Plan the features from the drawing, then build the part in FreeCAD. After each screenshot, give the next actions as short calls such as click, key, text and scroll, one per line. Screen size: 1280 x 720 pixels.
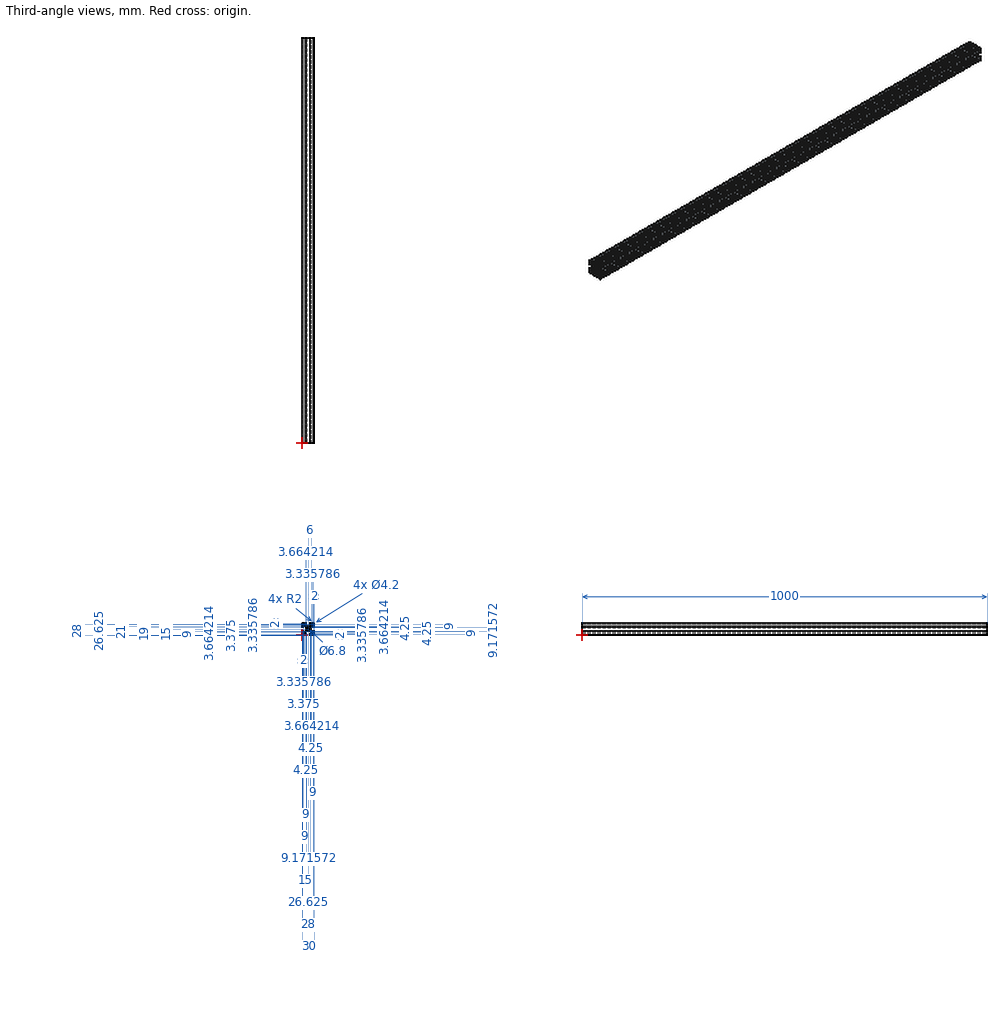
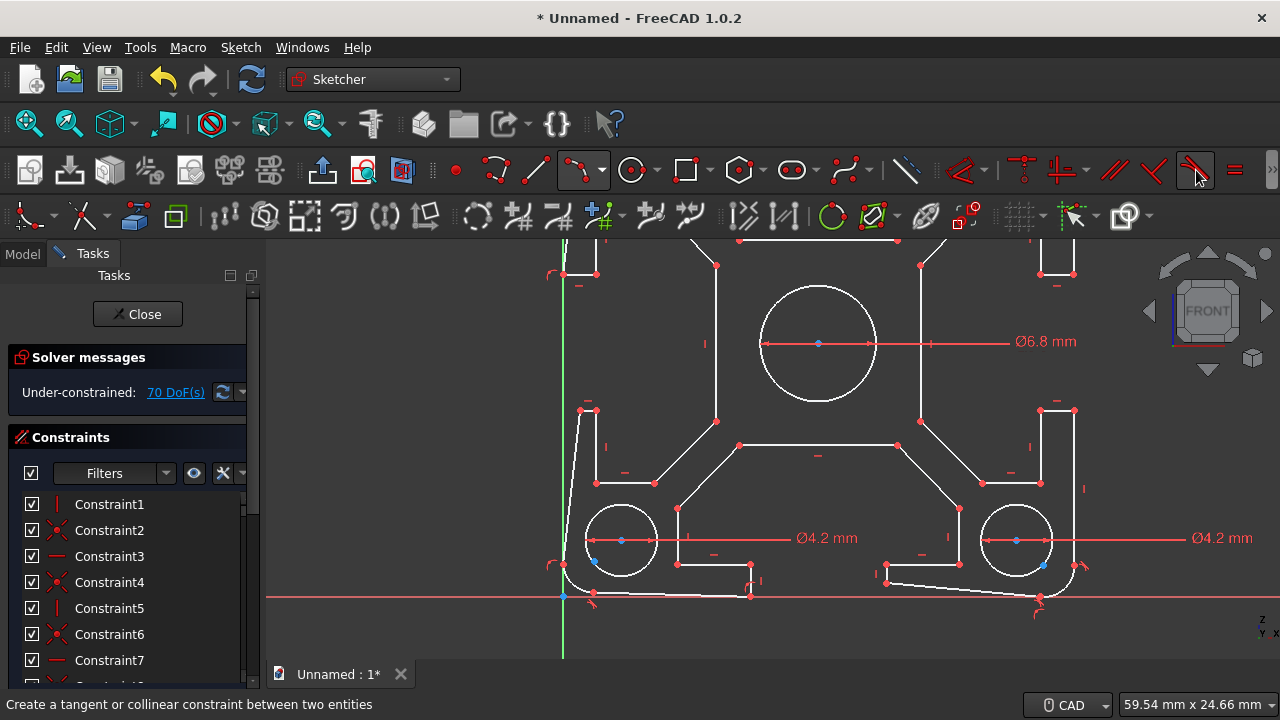
click(575, 457)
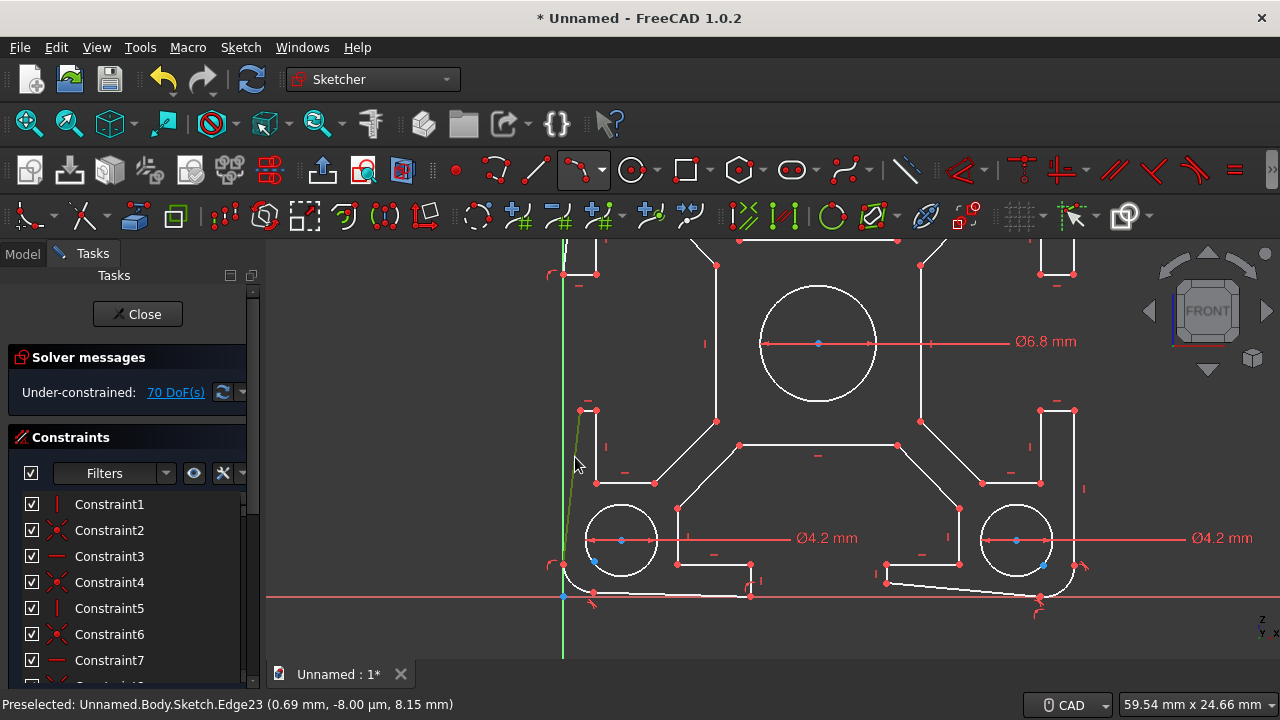
scroll(573, 584, up, 2)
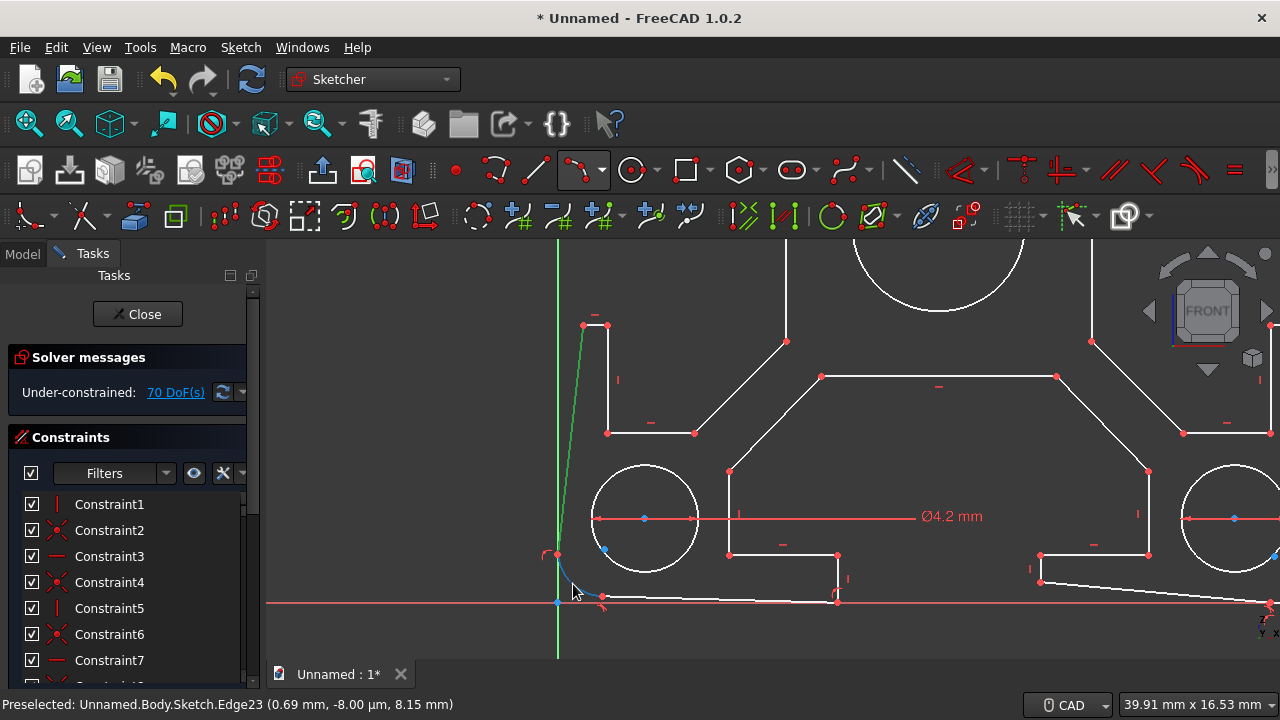
click(573, 584)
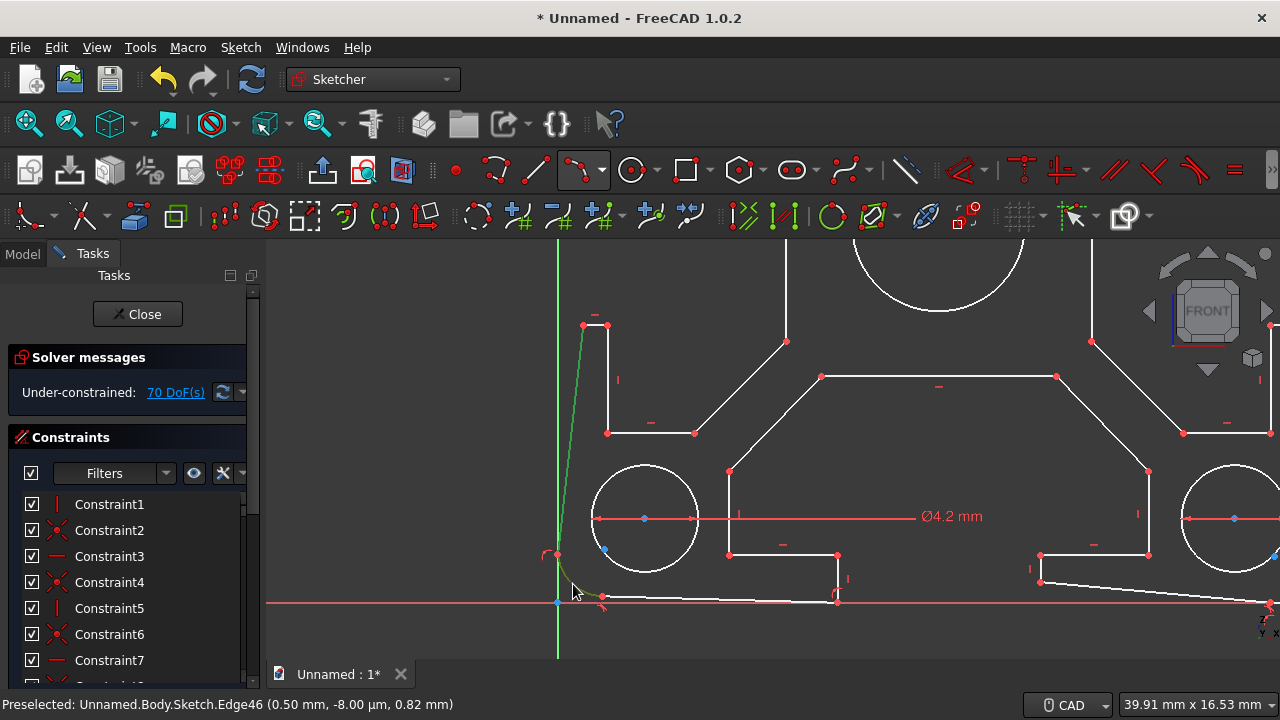
key(t)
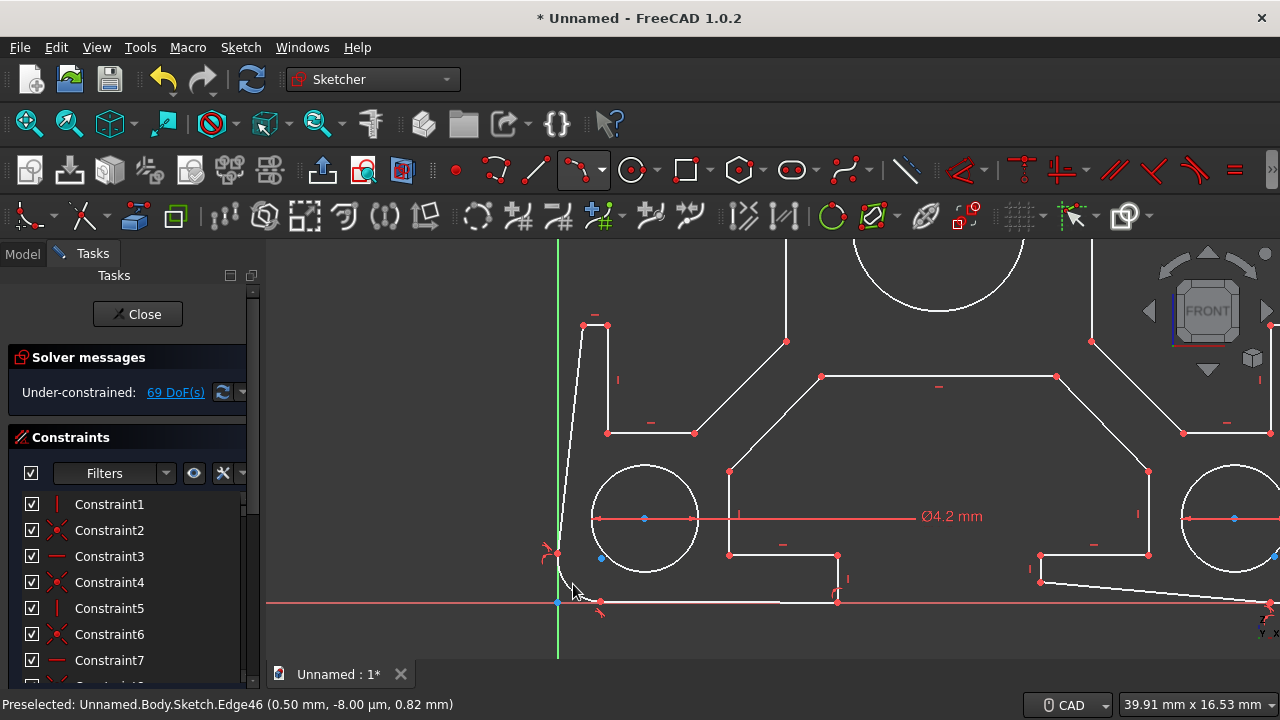
scroll(568, 581, down, 5)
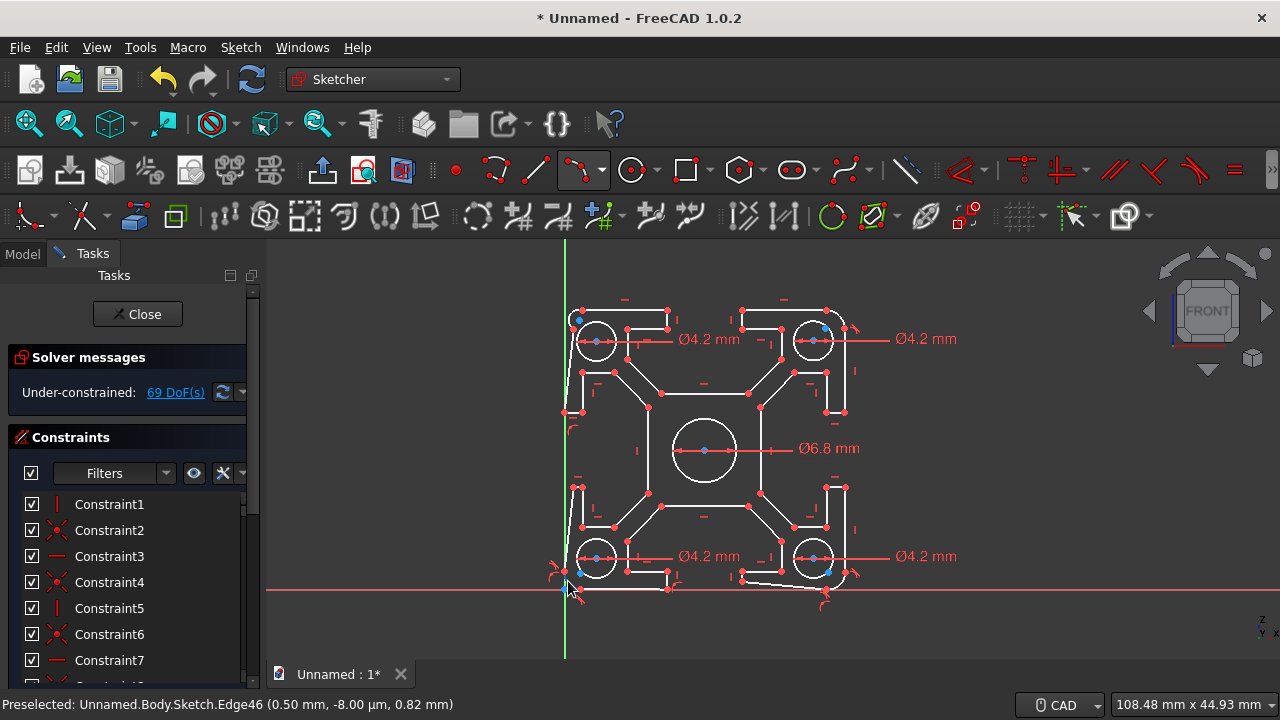
scroll(571, 354, up, 4)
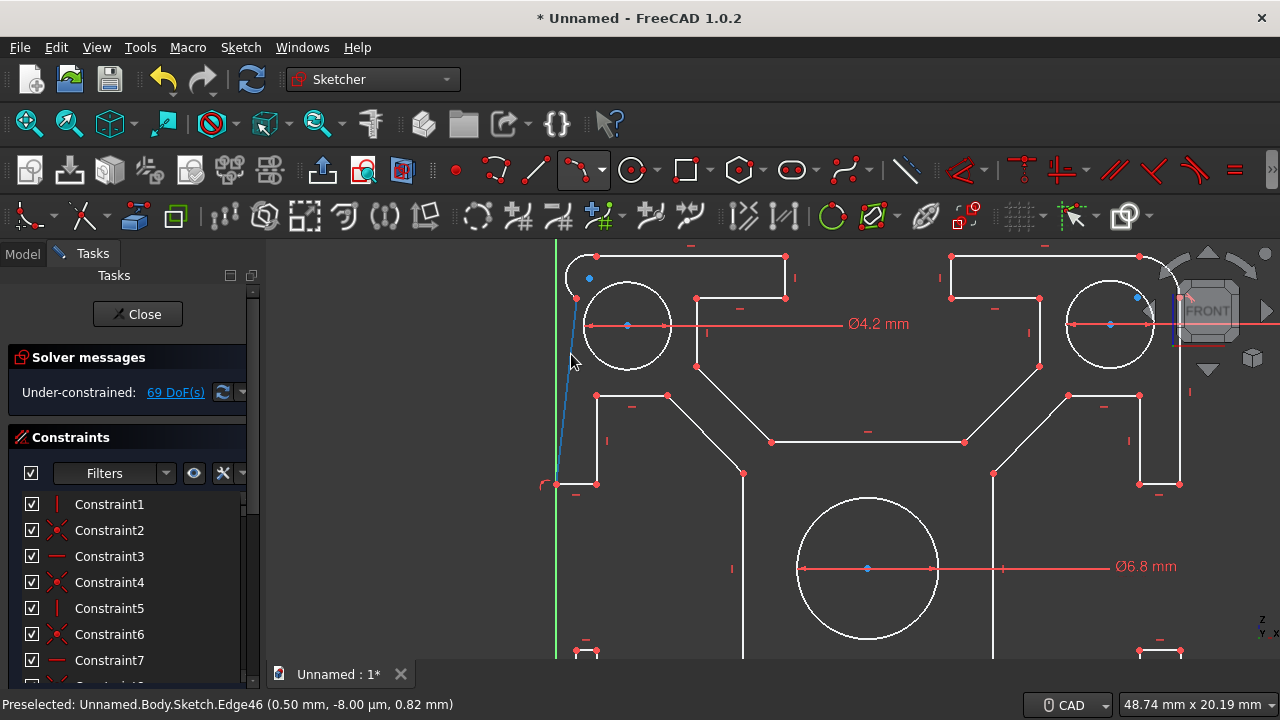
click(571, 354)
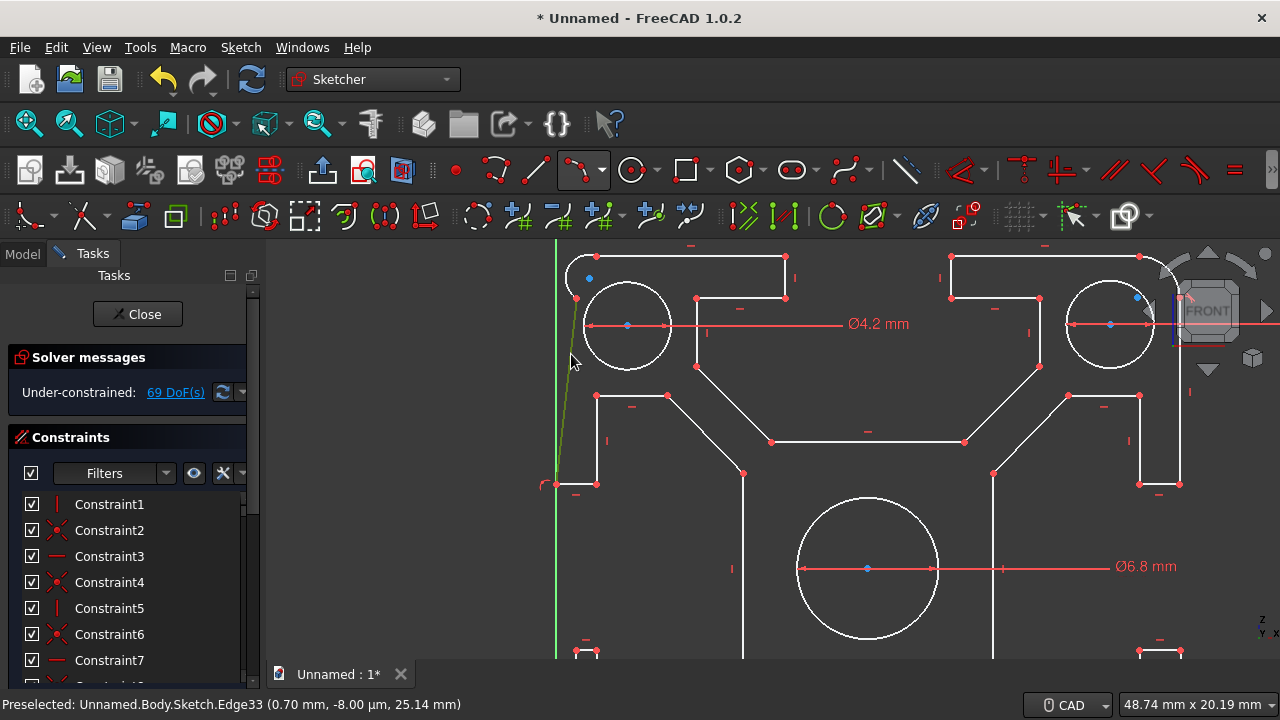
scroll(566, 282, up, 2)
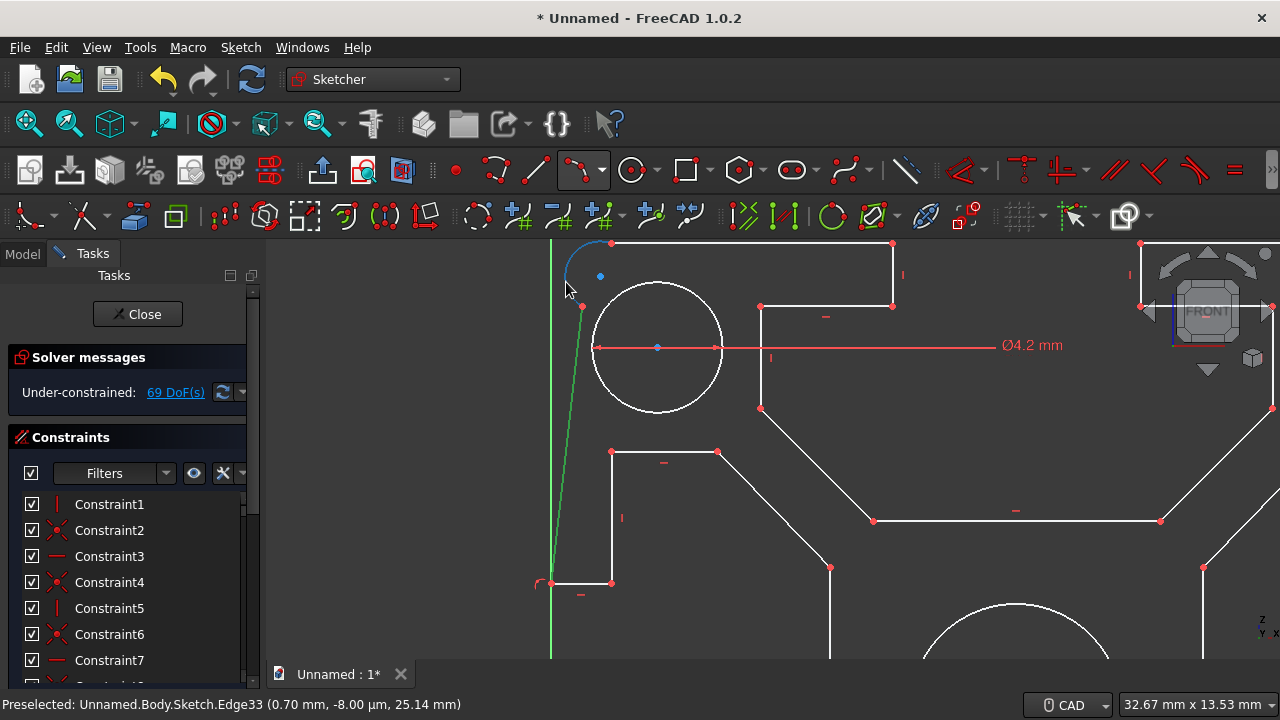
click(566, 281)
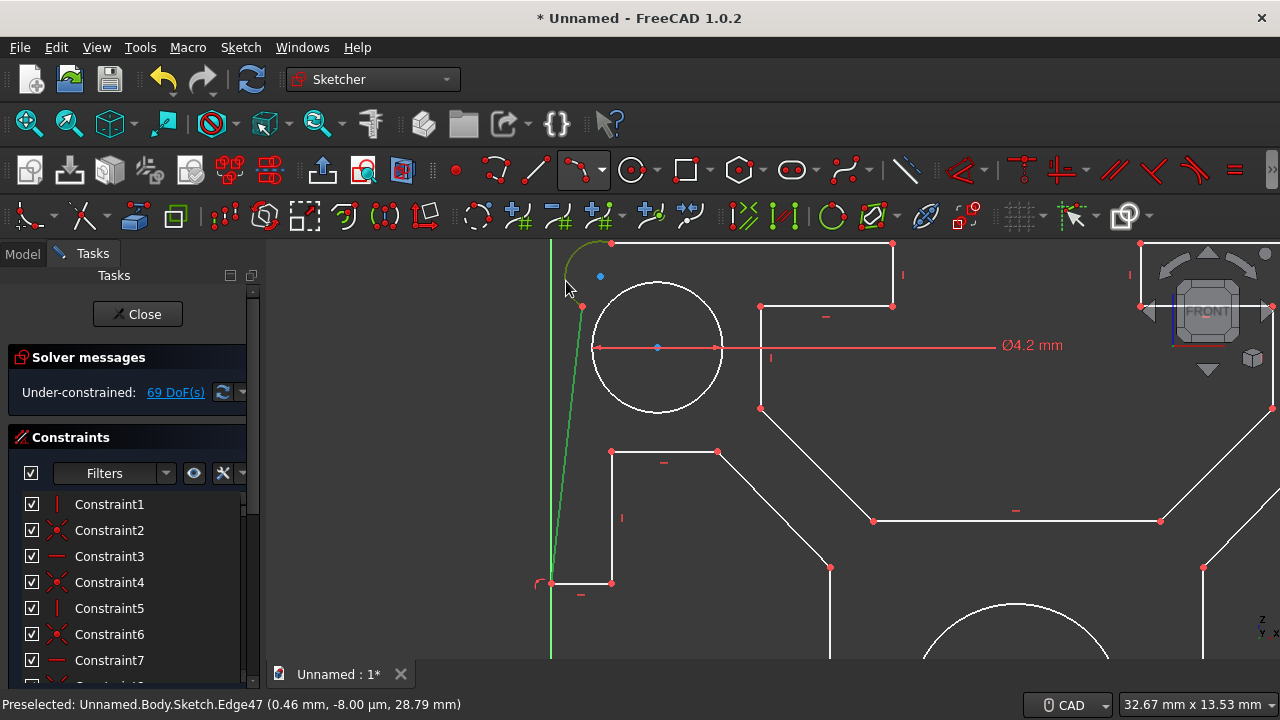
click(1196, 170)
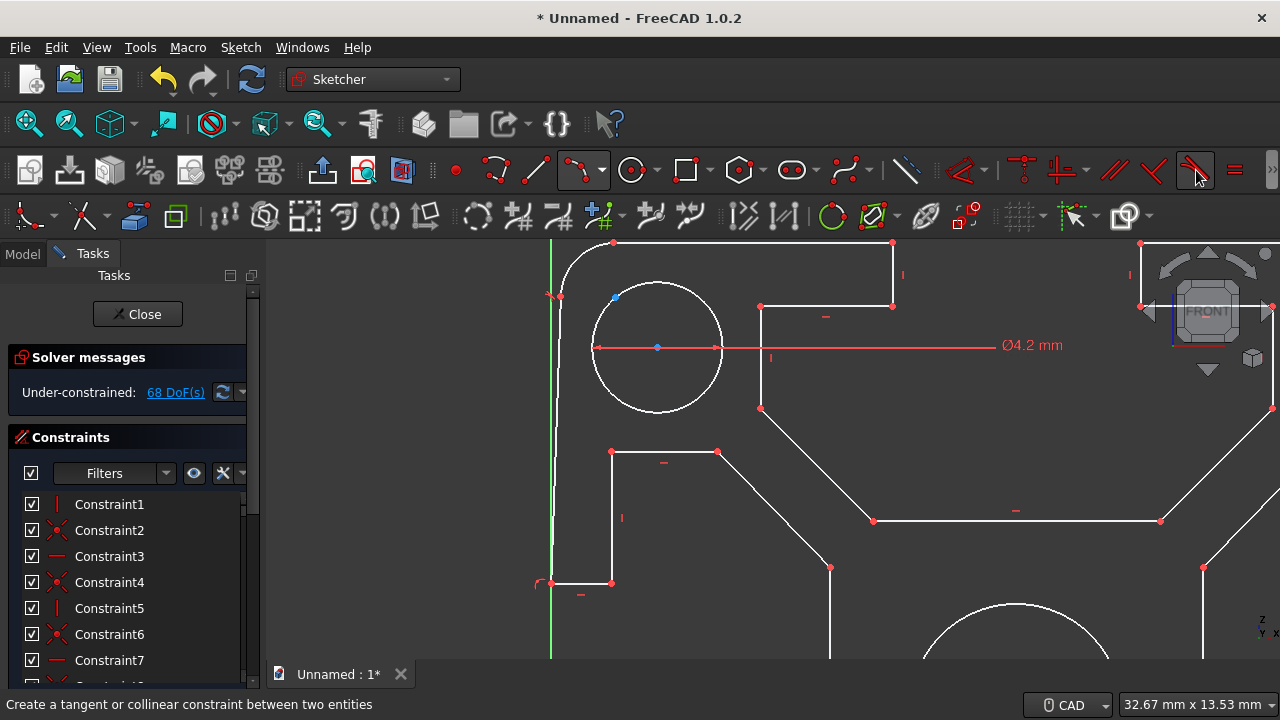
scroll(570, 339, down, 6)